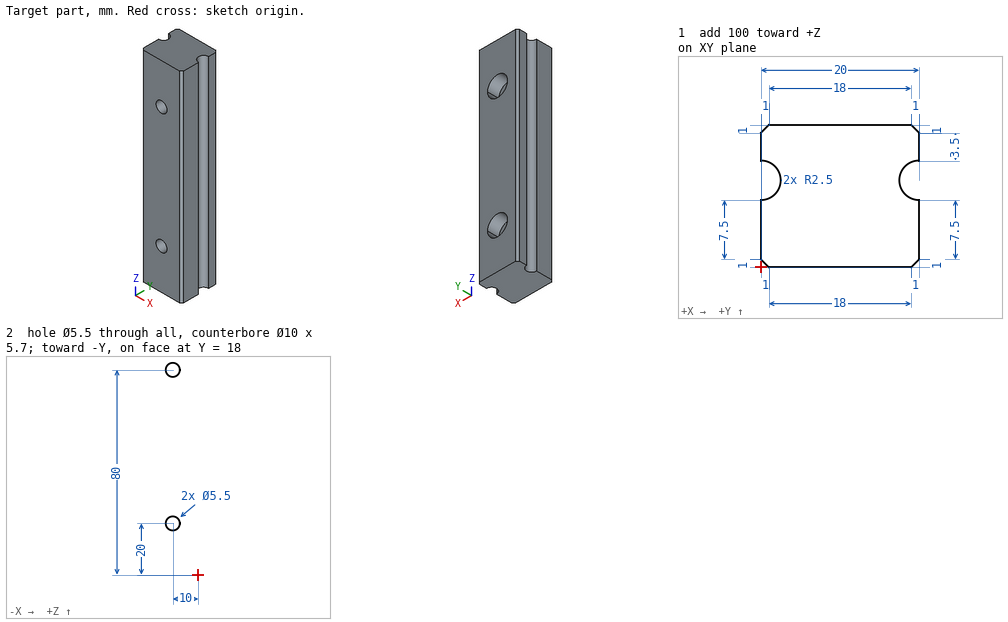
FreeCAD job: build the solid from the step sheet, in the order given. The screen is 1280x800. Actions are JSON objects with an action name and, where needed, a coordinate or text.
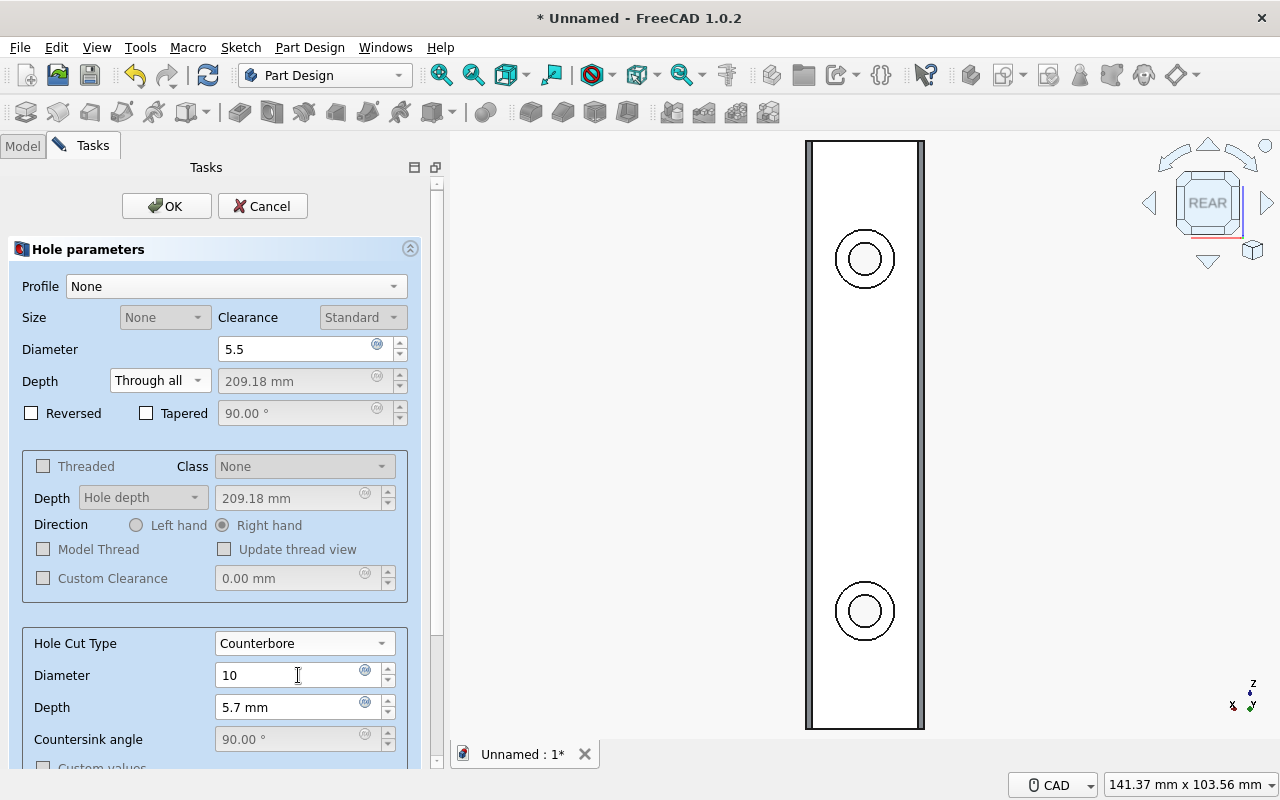
{"action": "left_click", "coordinate": [167, 206]}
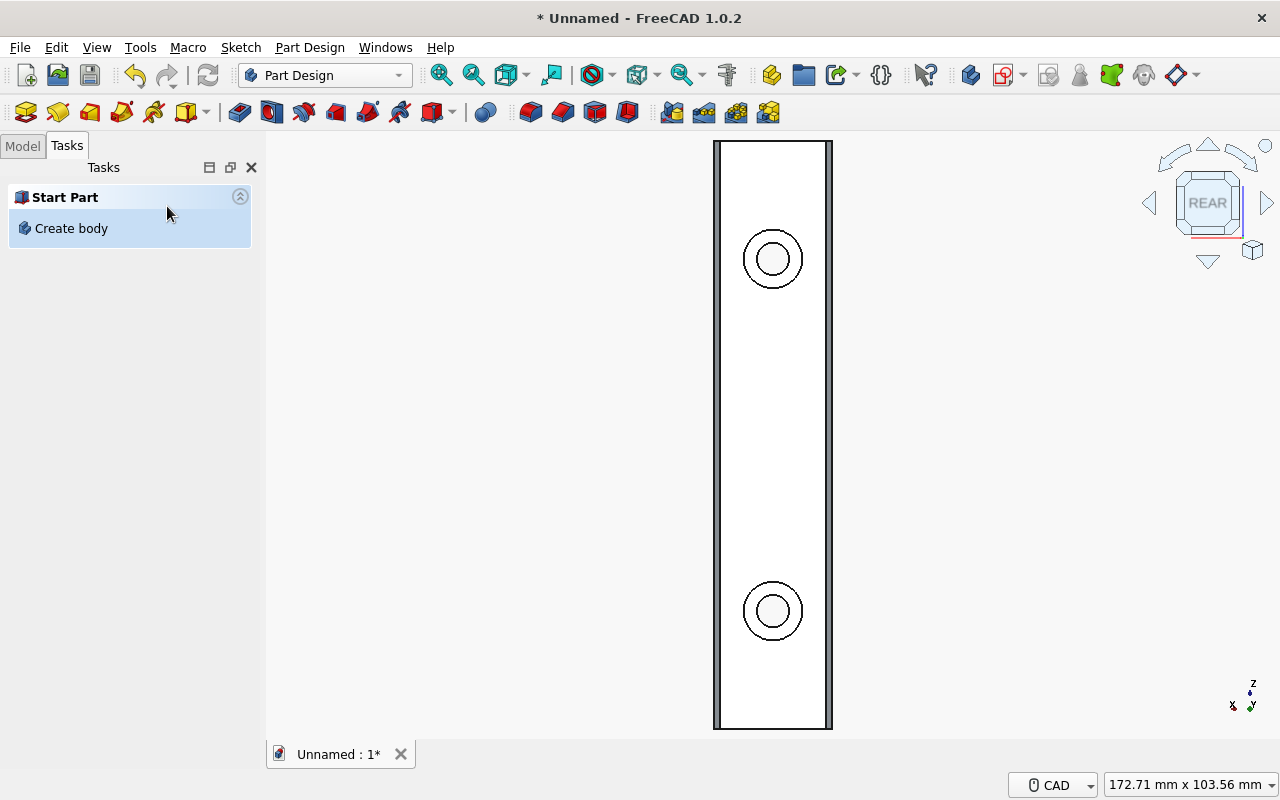
{"action": "key", "text": "0"}